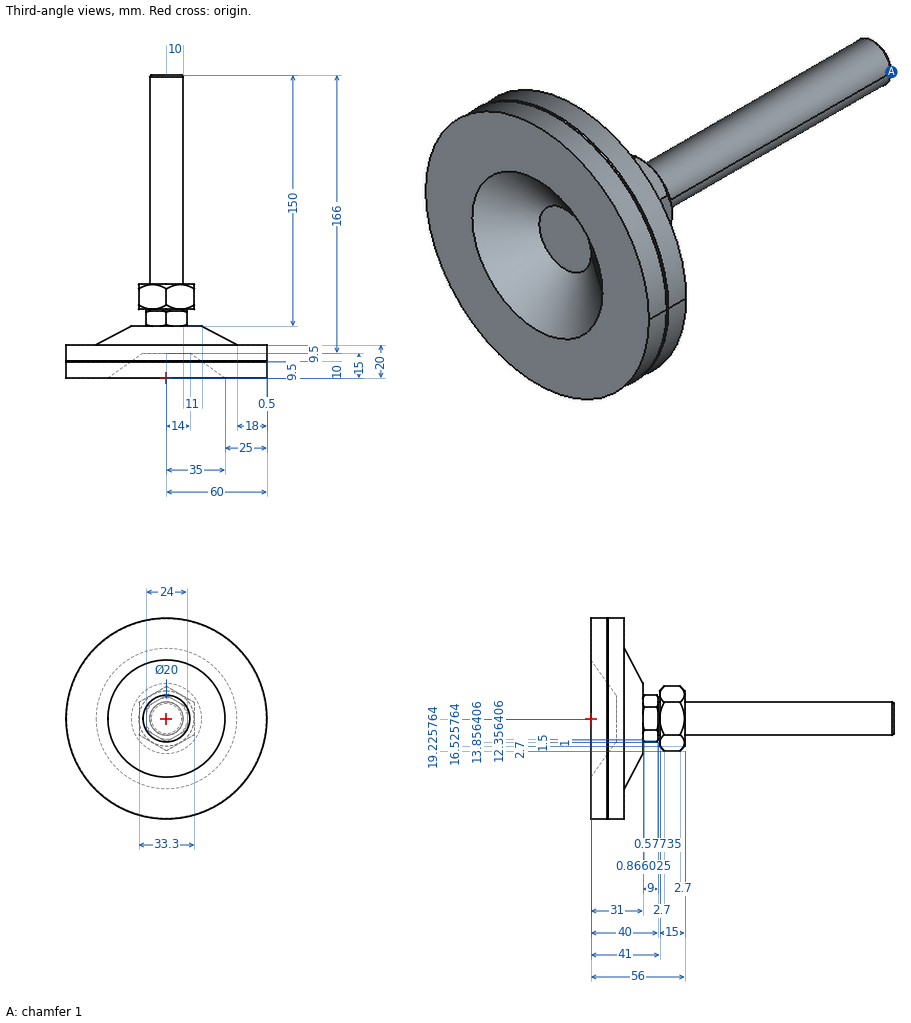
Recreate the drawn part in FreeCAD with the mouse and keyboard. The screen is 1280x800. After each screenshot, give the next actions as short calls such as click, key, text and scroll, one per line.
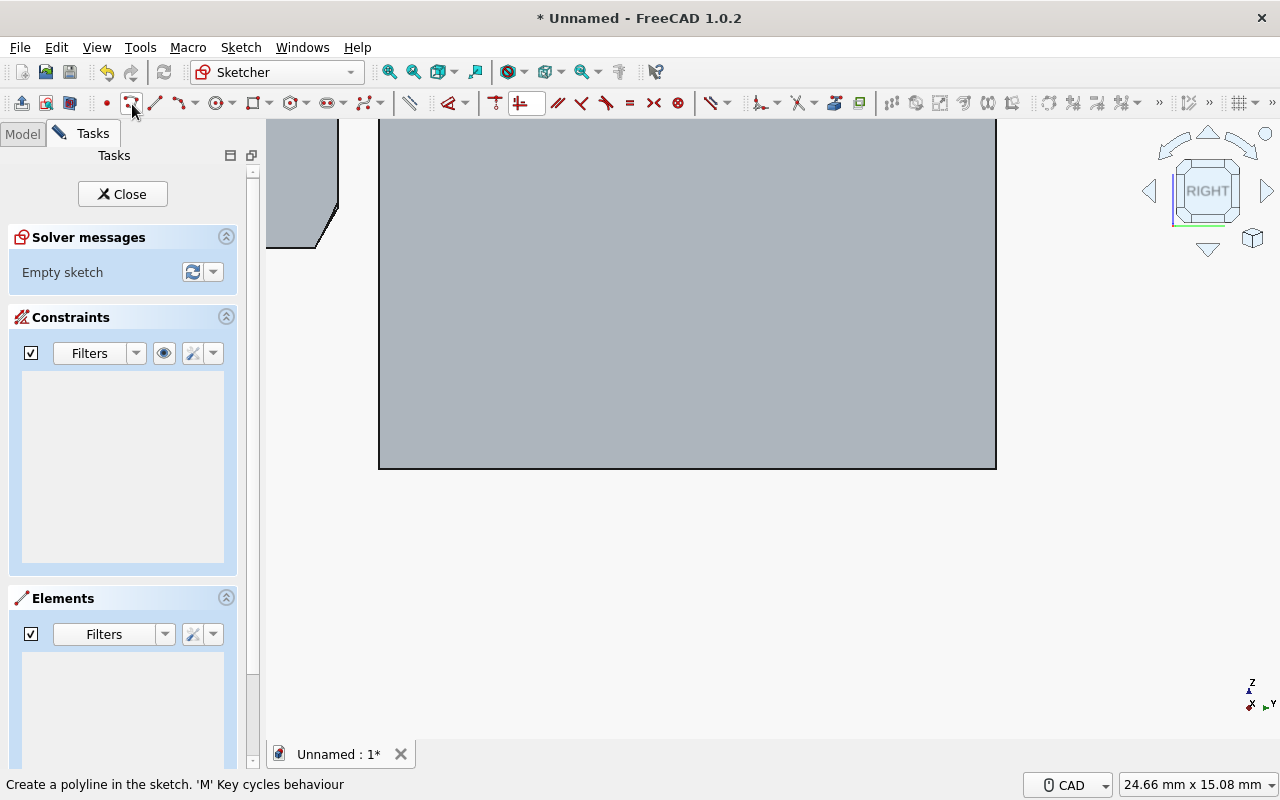
click(885, 469)
click(996, 469)
click(996, 358)
click(885, 470)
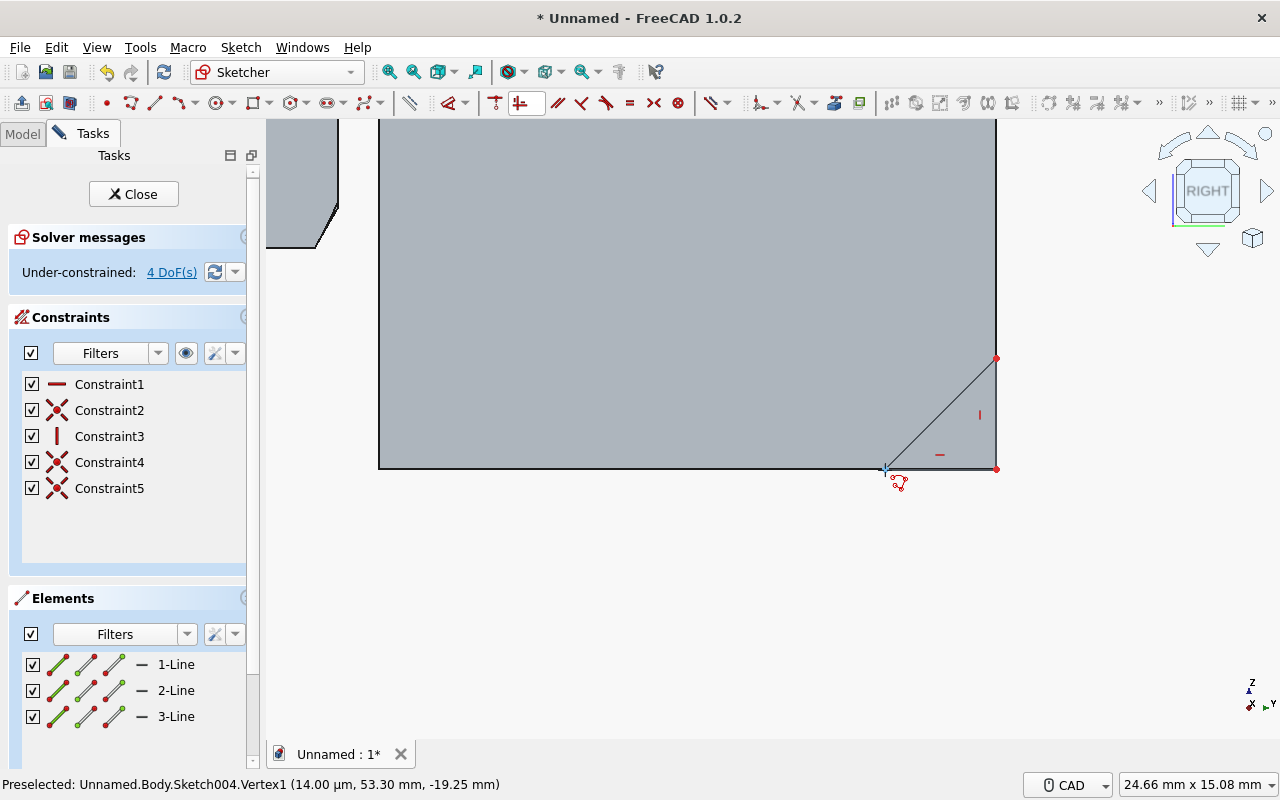
click(379, 358)
click(379, 469)
click(490, 469)
click(379, 359)
key(Escape)
key(Escape)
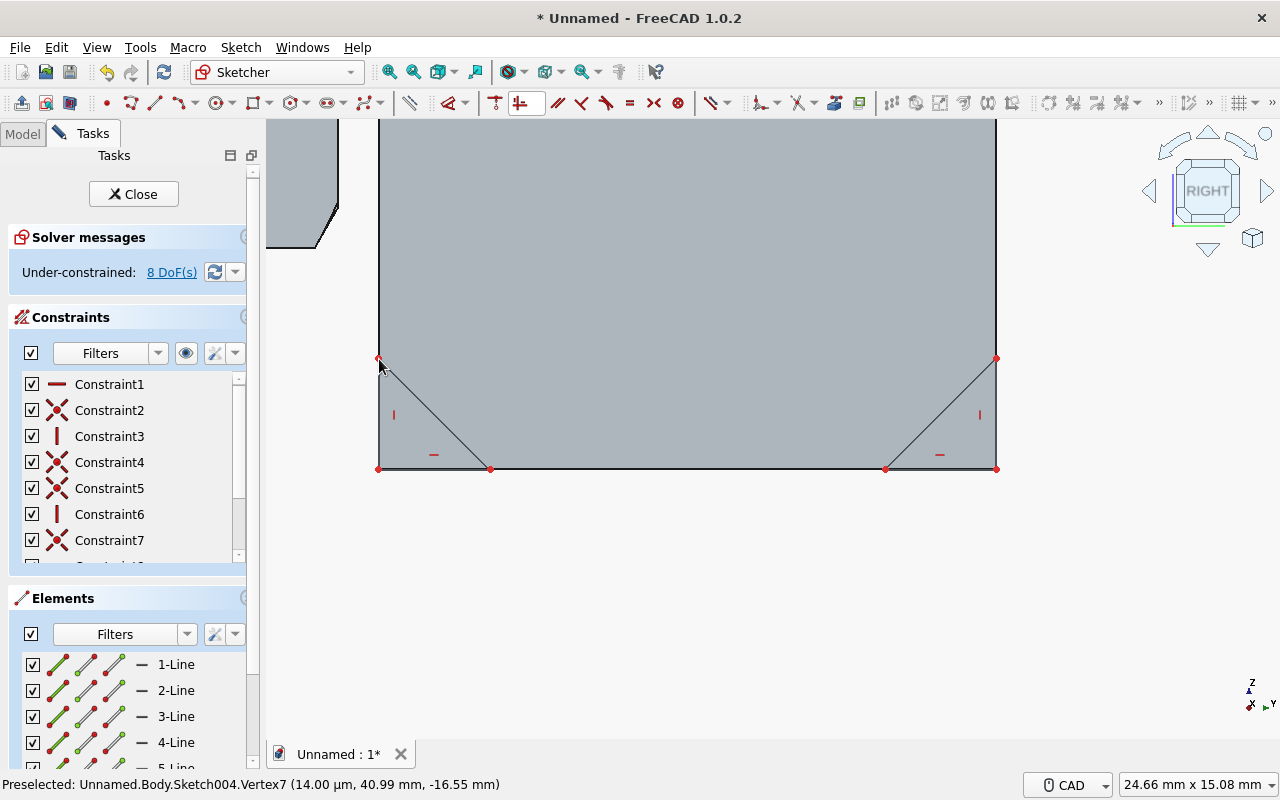
click(448, 104)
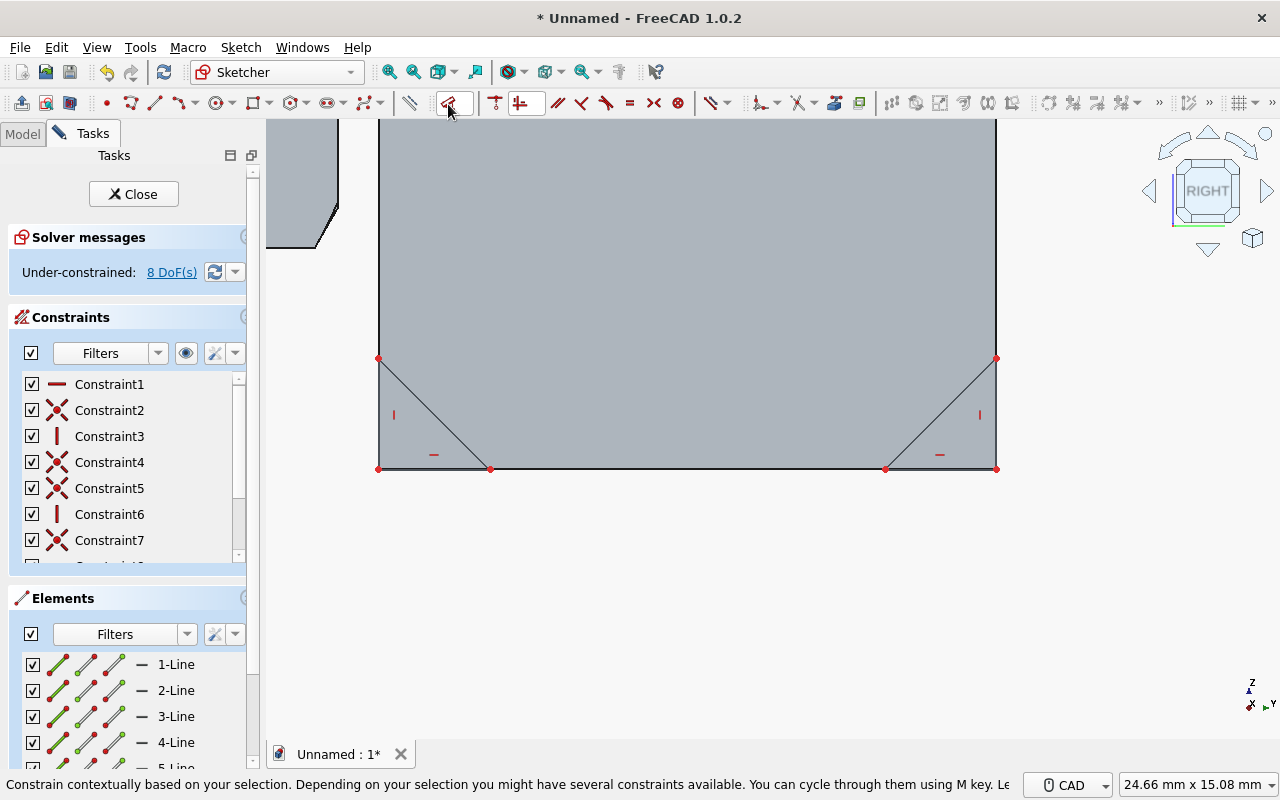
click(918, 470)
click(941, 504)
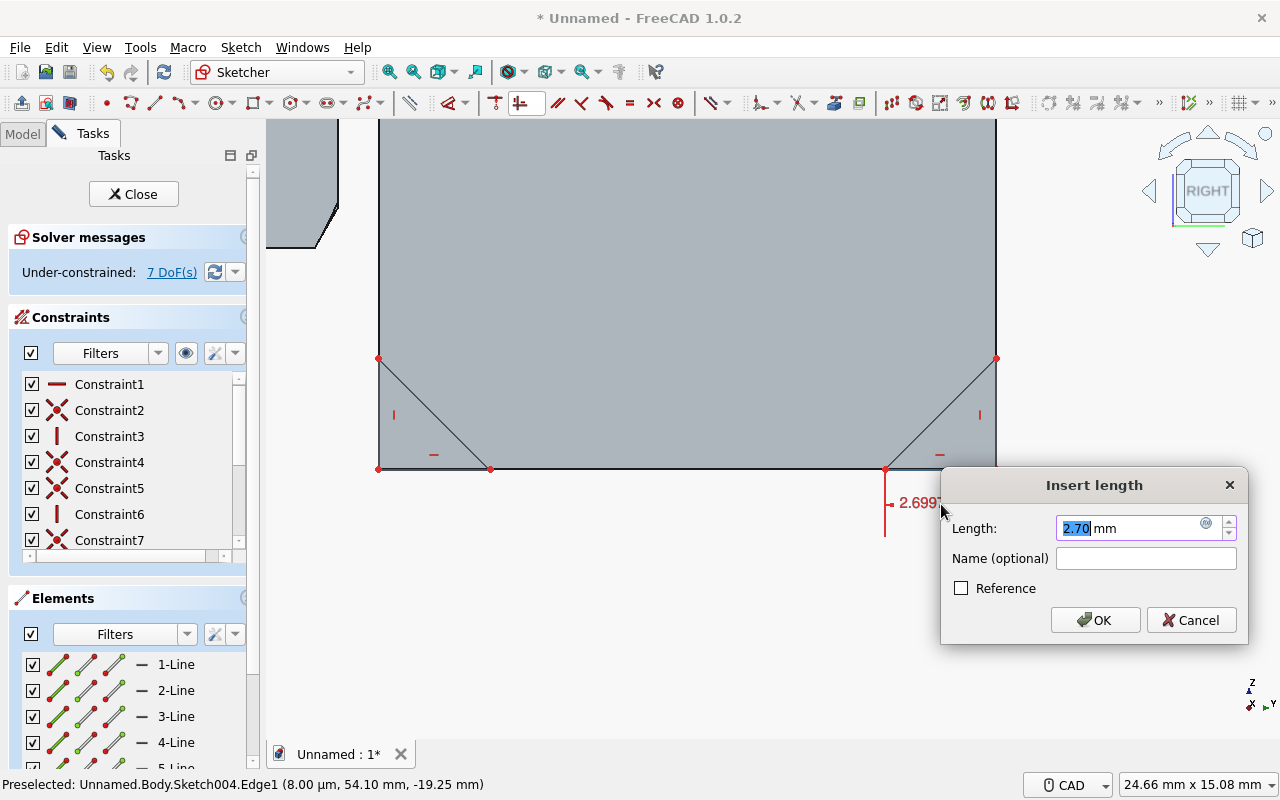
text(2.7)
key(Return)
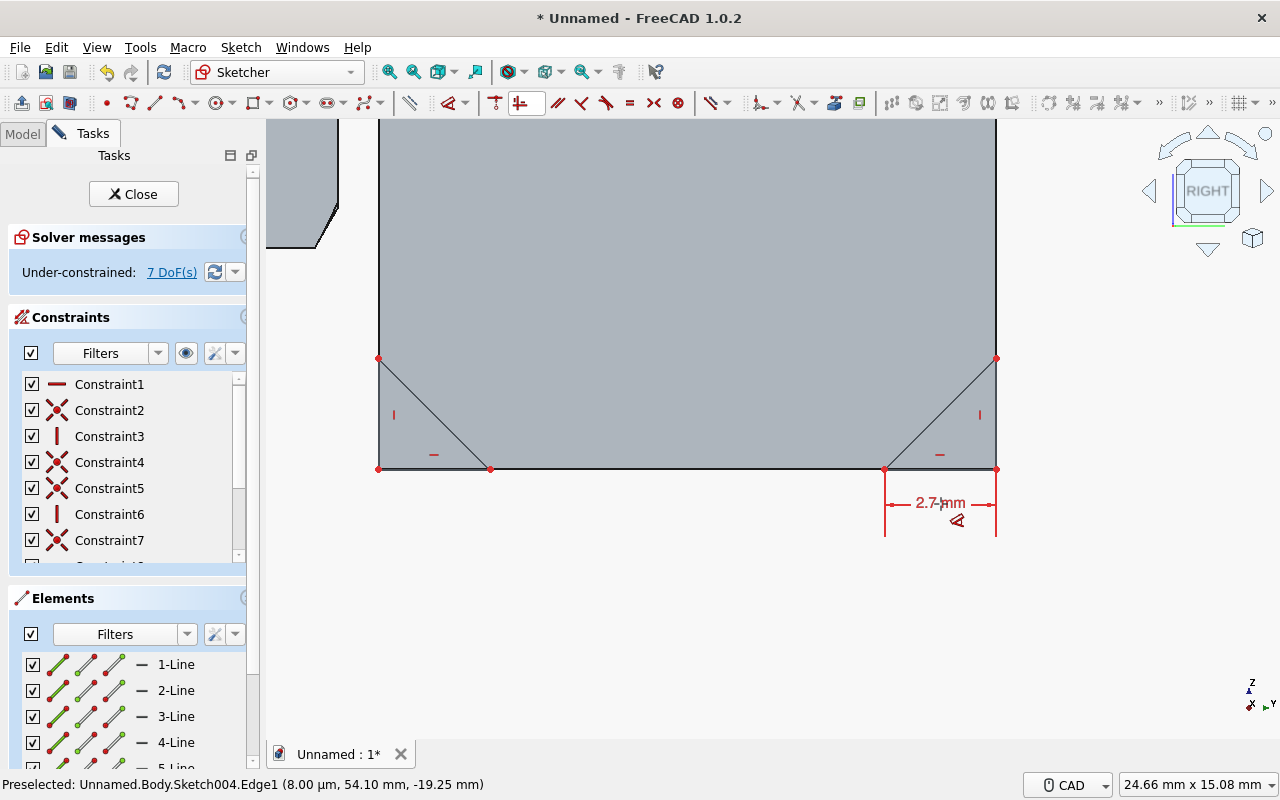
click(996, 437)
click(1030, 414)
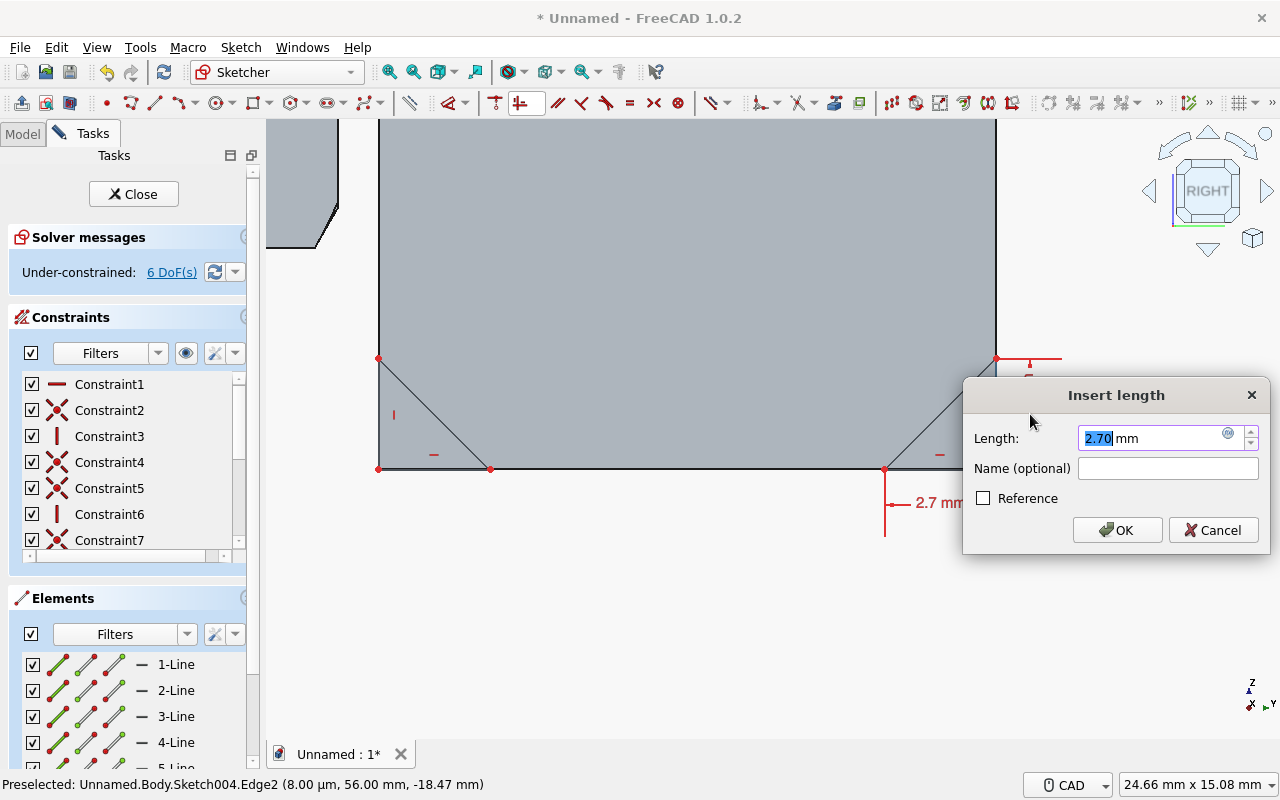
text(2.7)
key(Return)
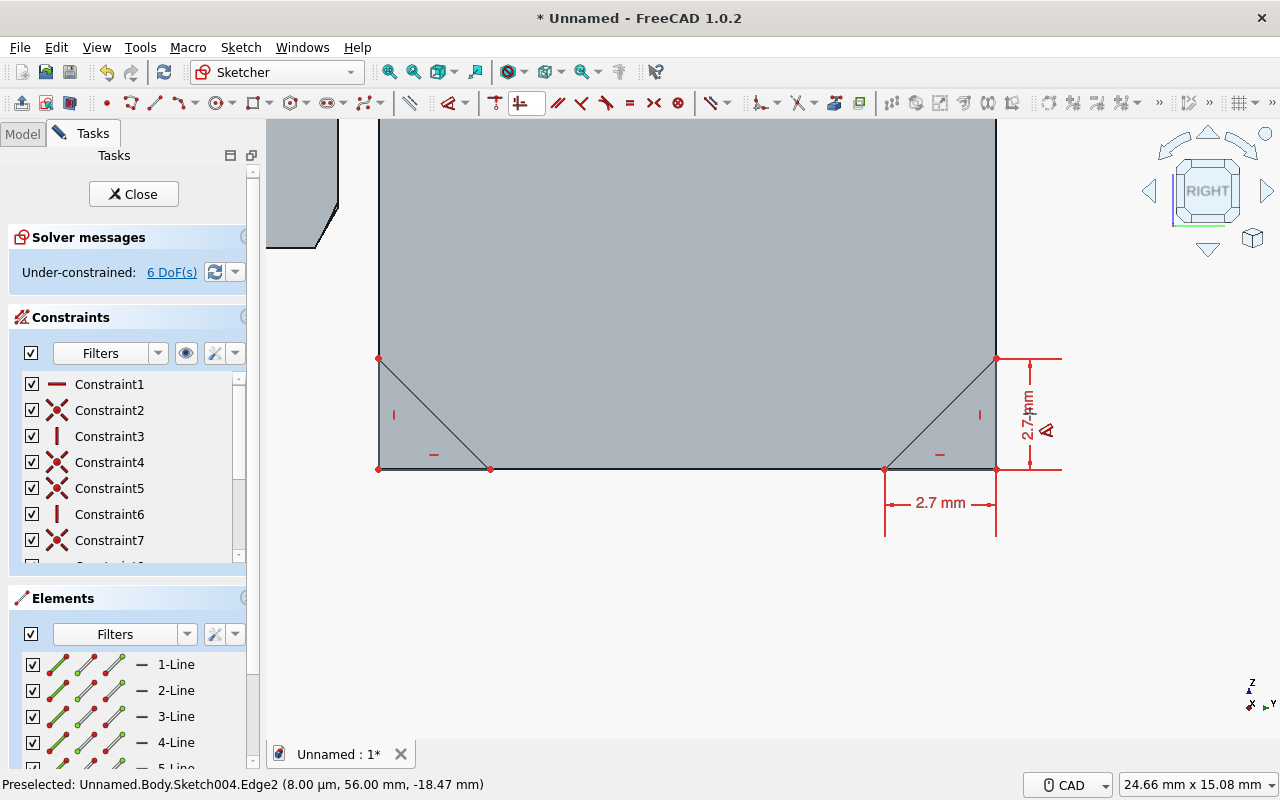
click(379, 392)
click(345, 414)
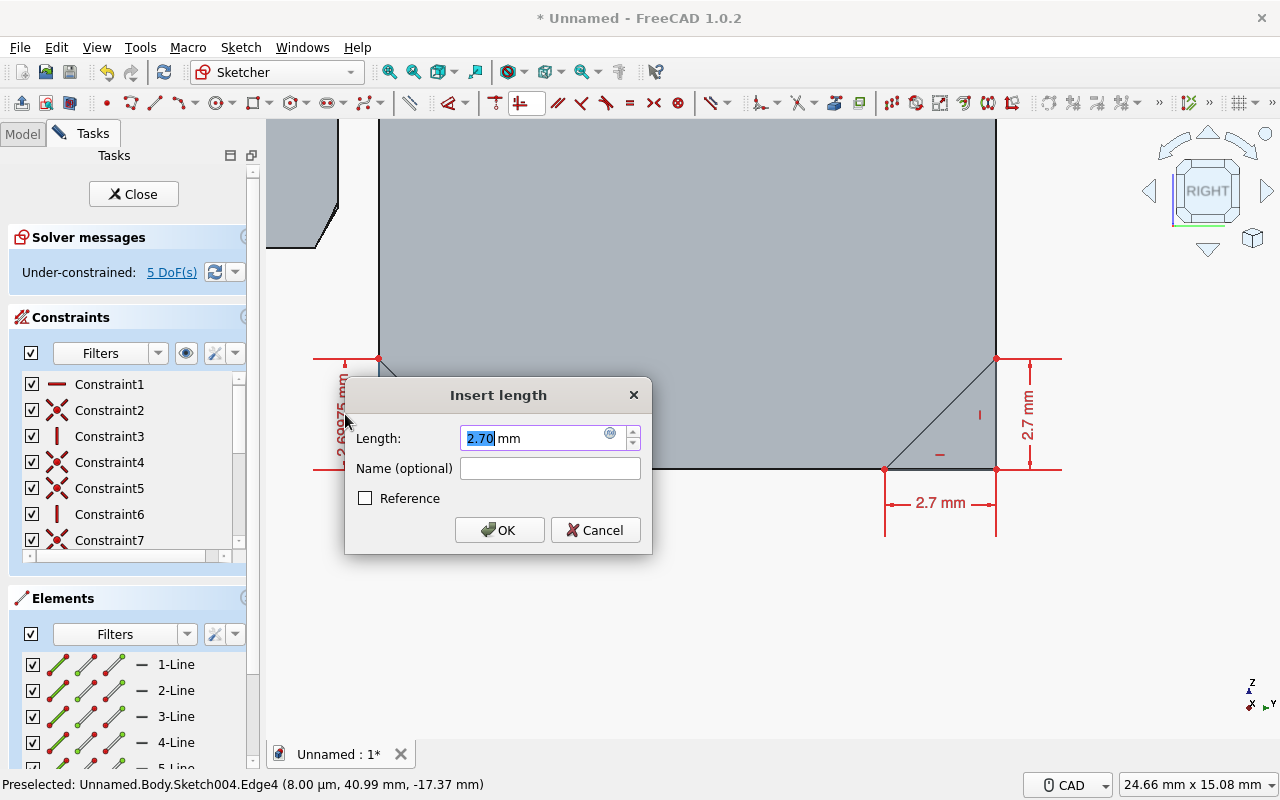
text(2.7)
key(Return)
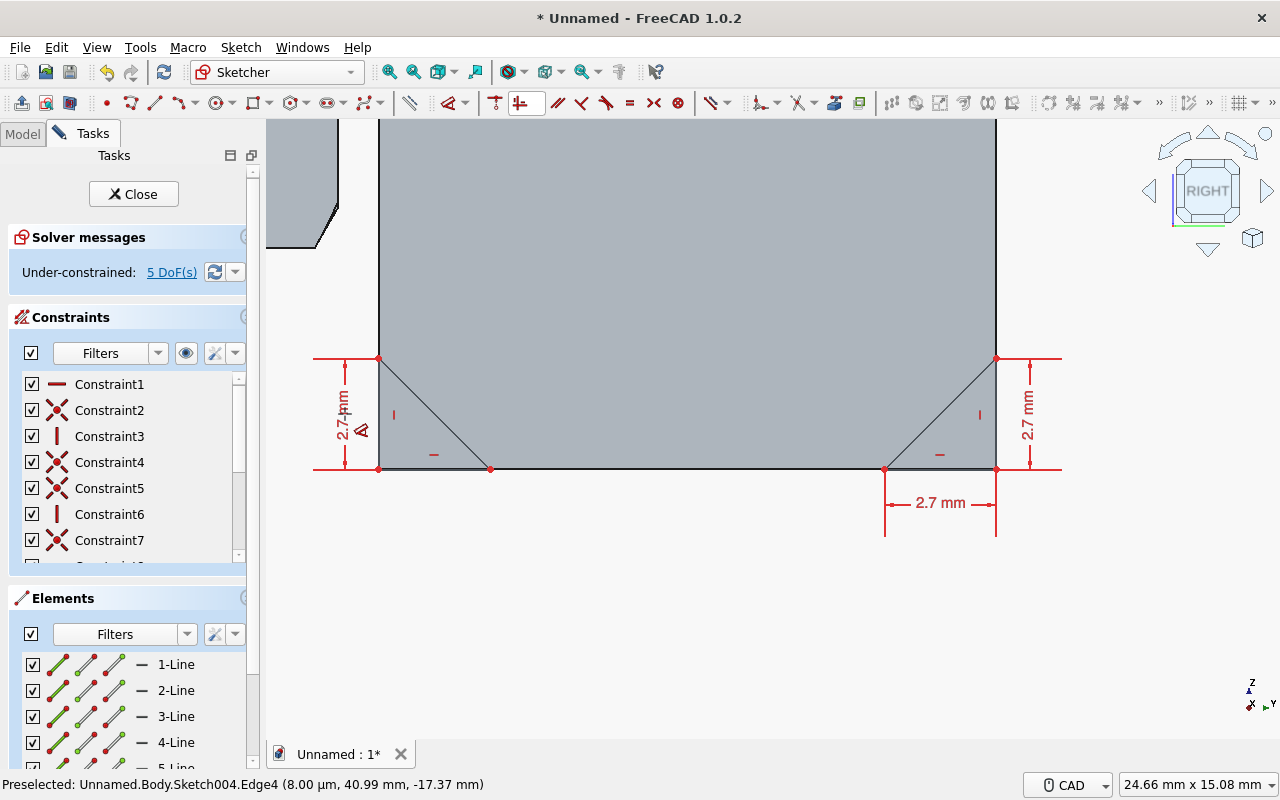
click(412, 470)
click(434, 504)